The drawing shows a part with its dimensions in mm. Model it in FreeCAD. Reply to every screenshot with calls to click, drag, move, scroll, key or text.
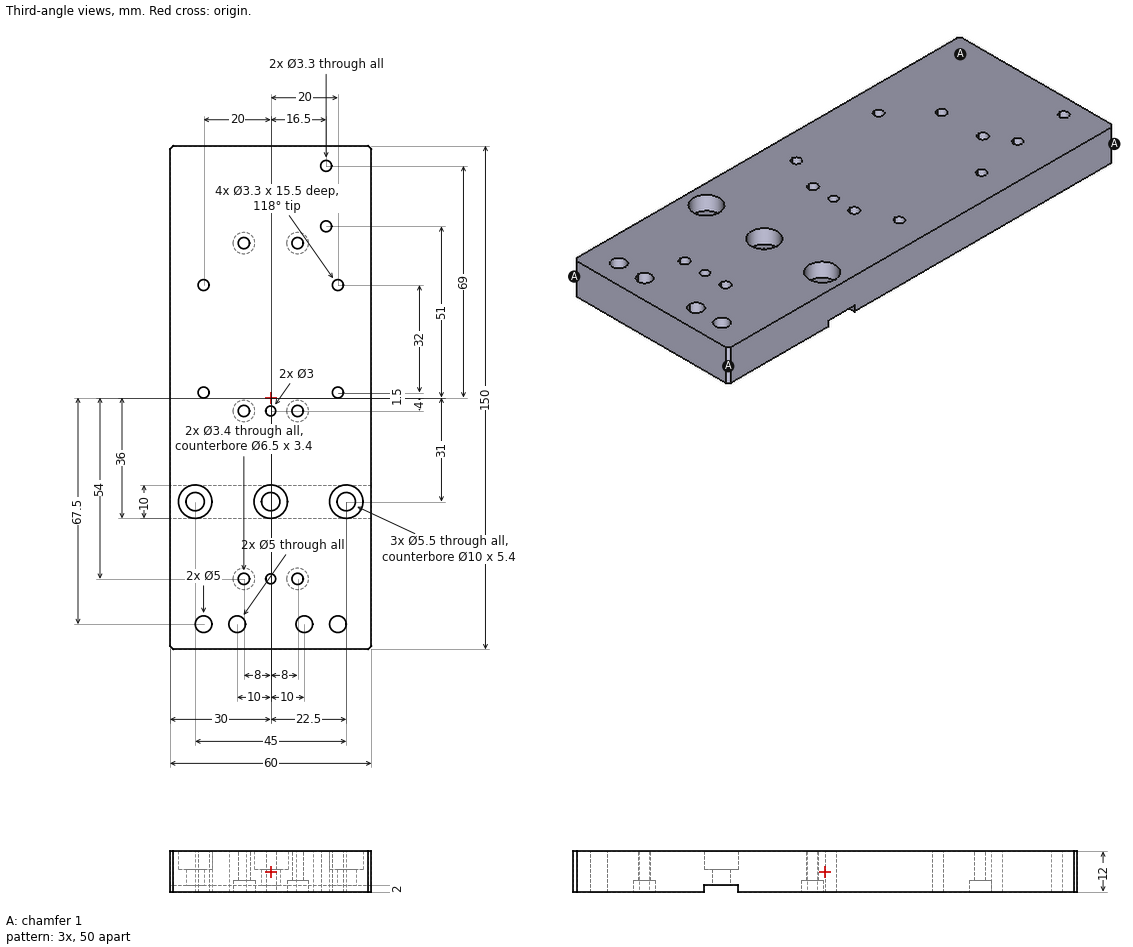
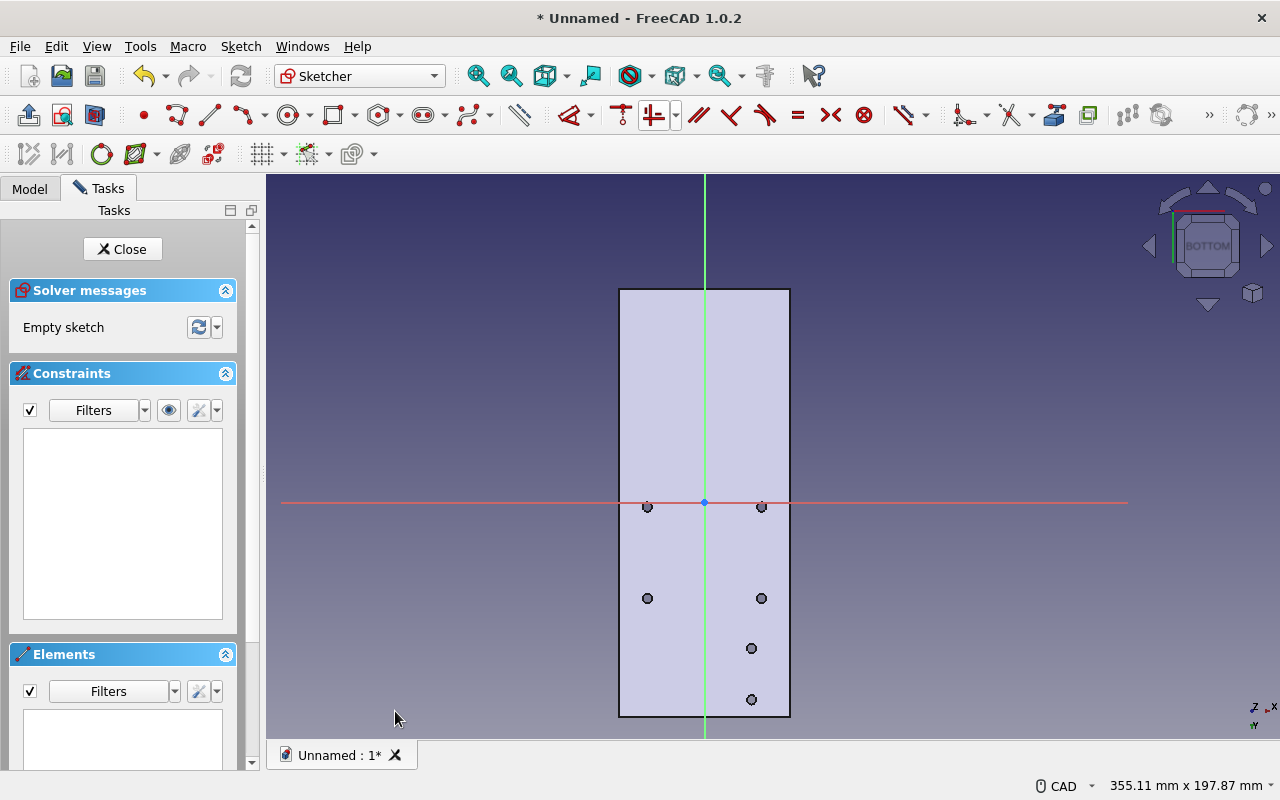
scroll(705, 338, up, 3)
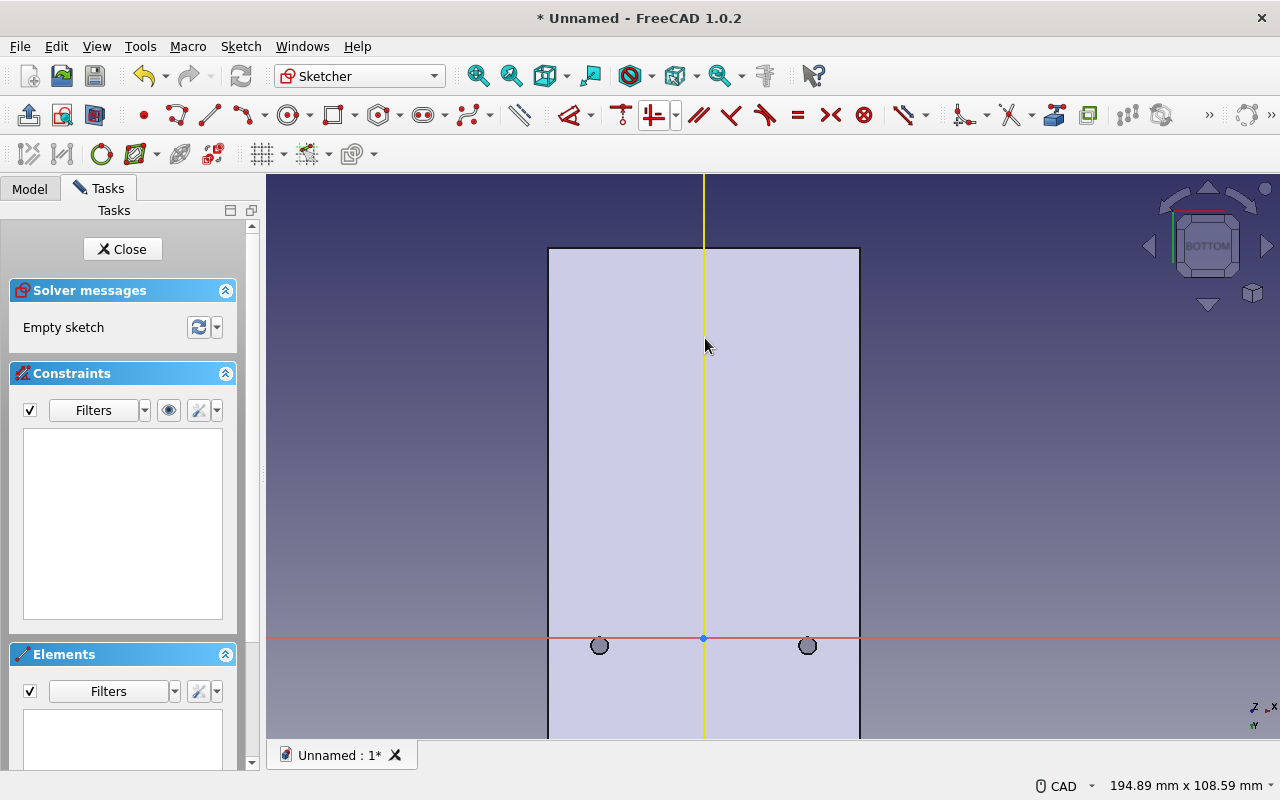
click(288, 116)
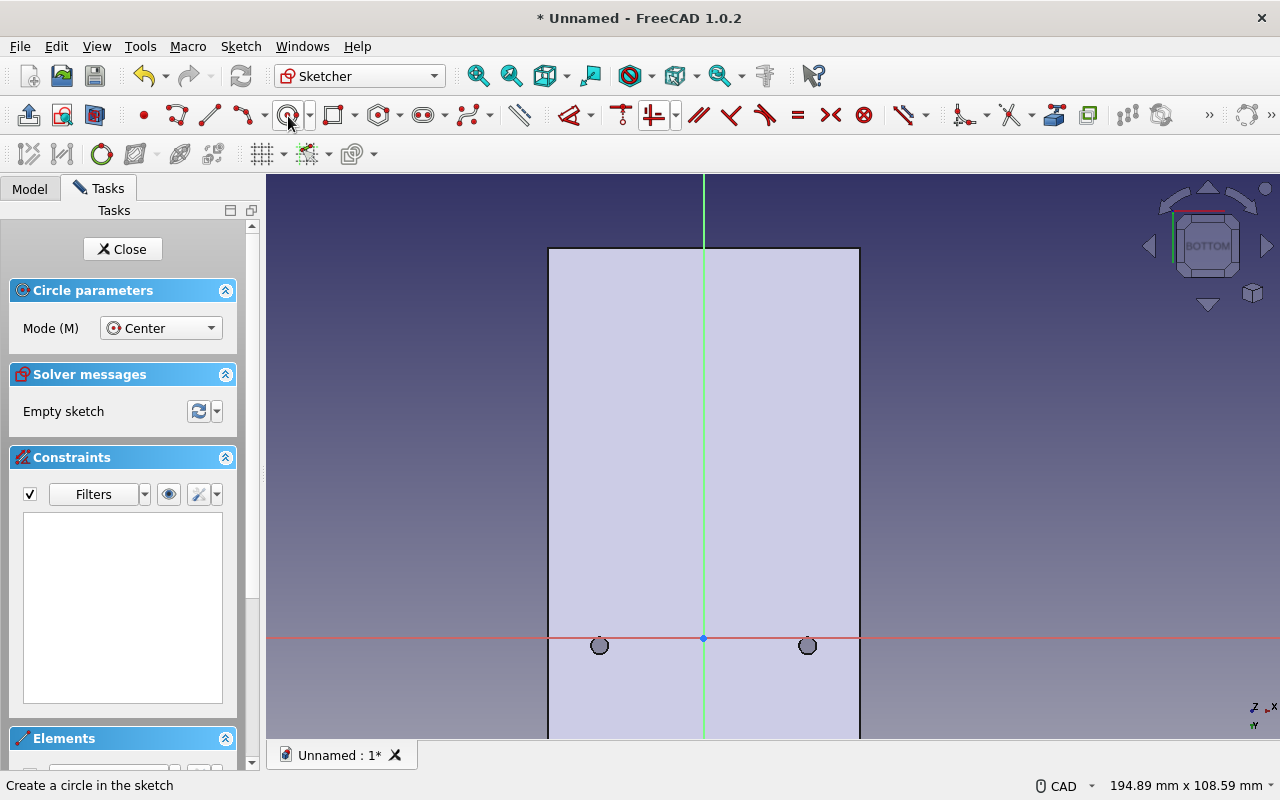
scroll(600, 287, up, 3)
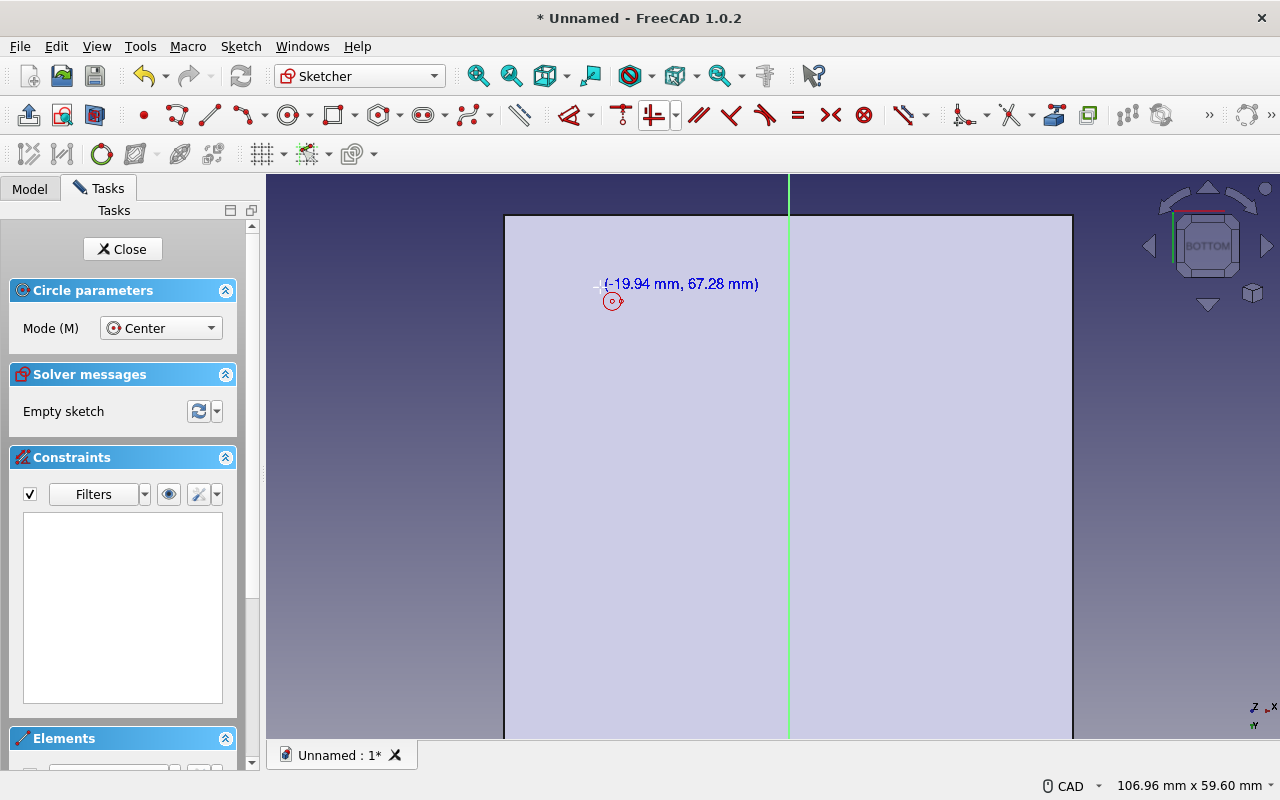
click(599, 287)
click(616, 270)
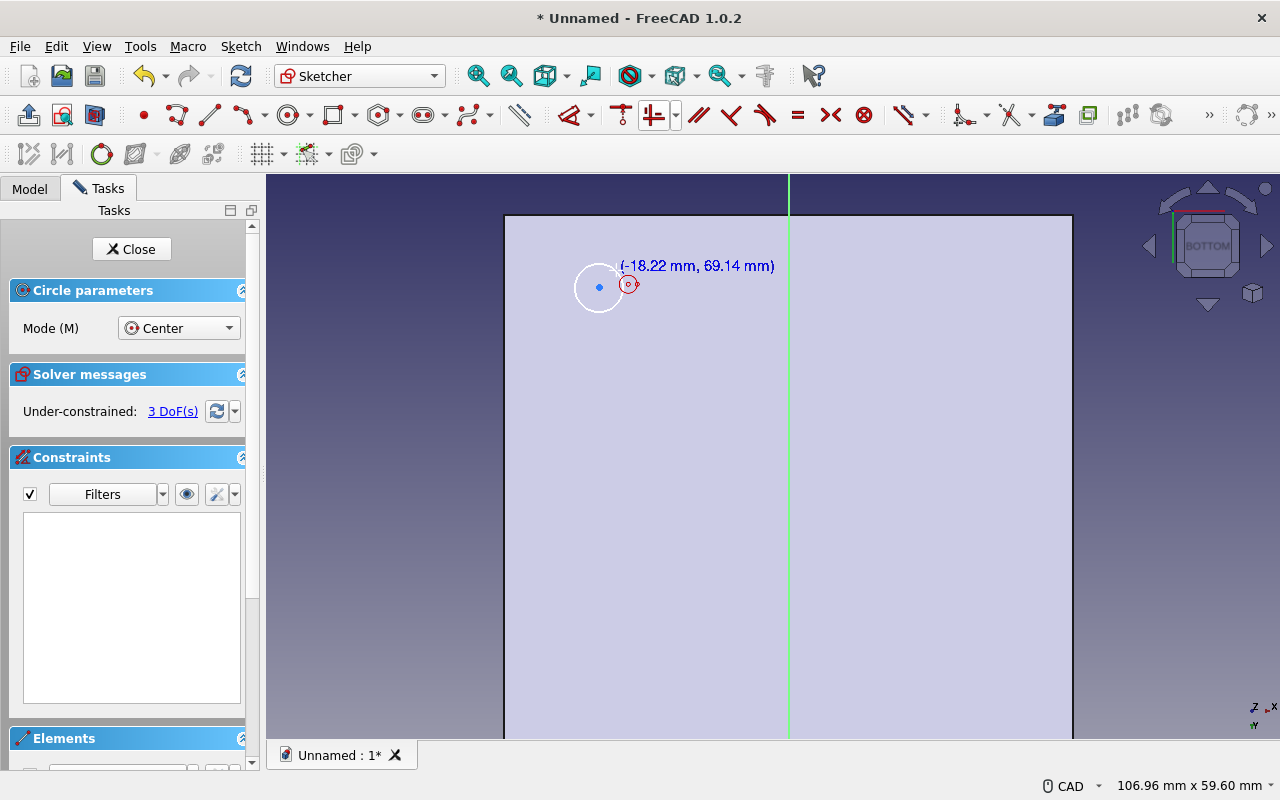
click(978, 287)
click(995, 270)
key(Escape)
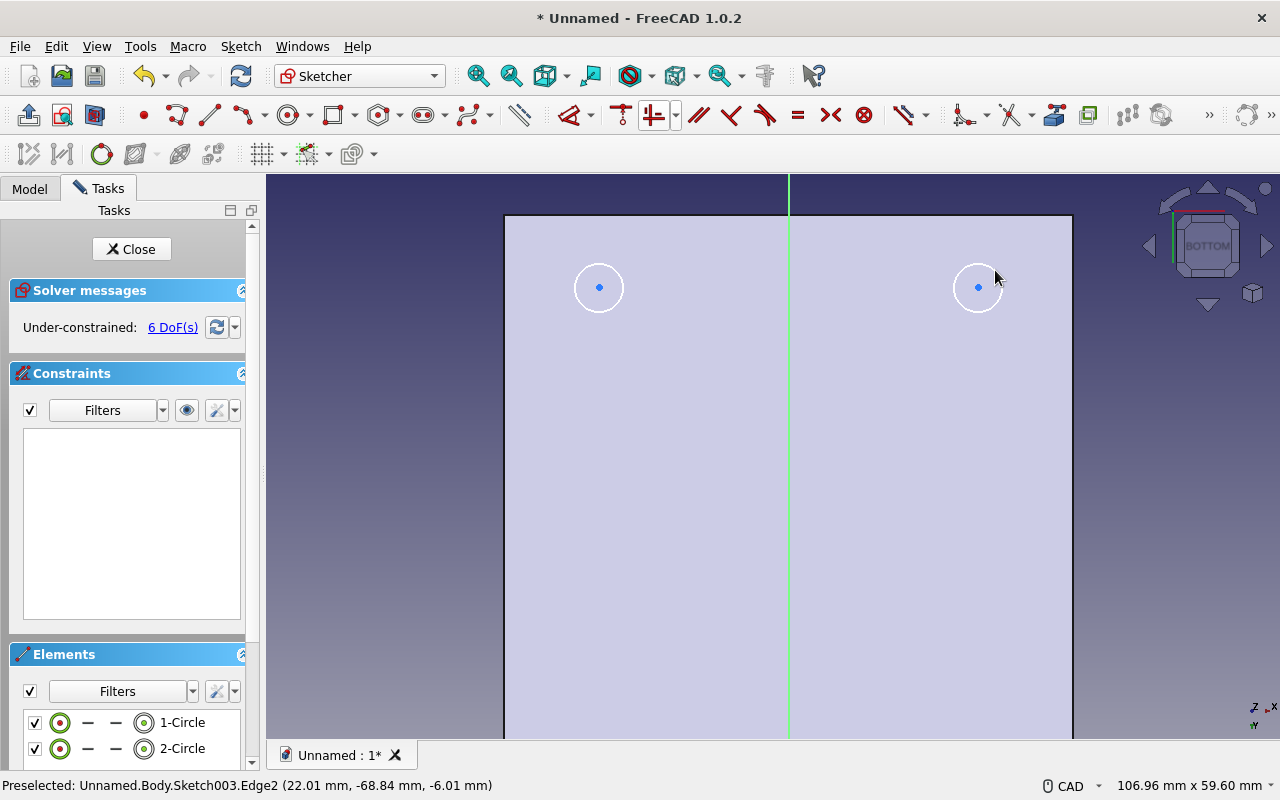
click(616, 271)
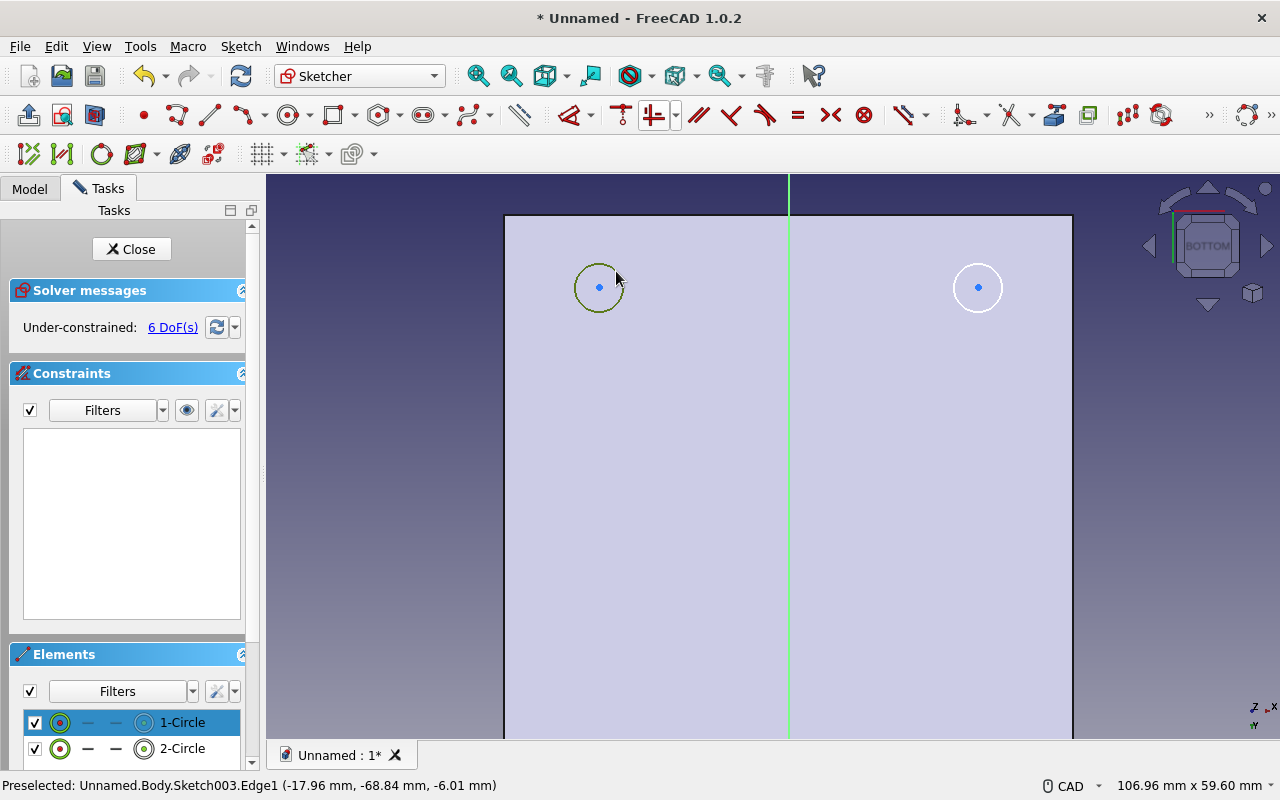
click(995, 271)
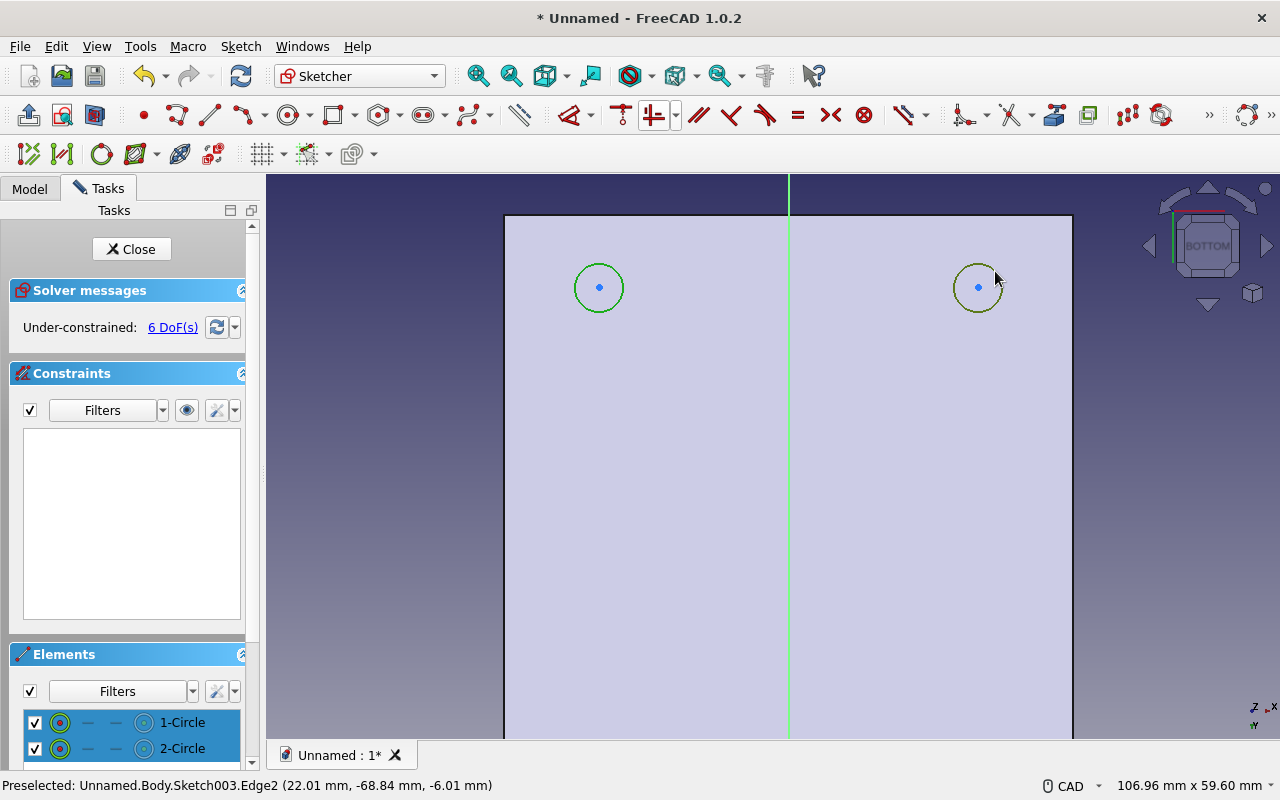
click(798, 116)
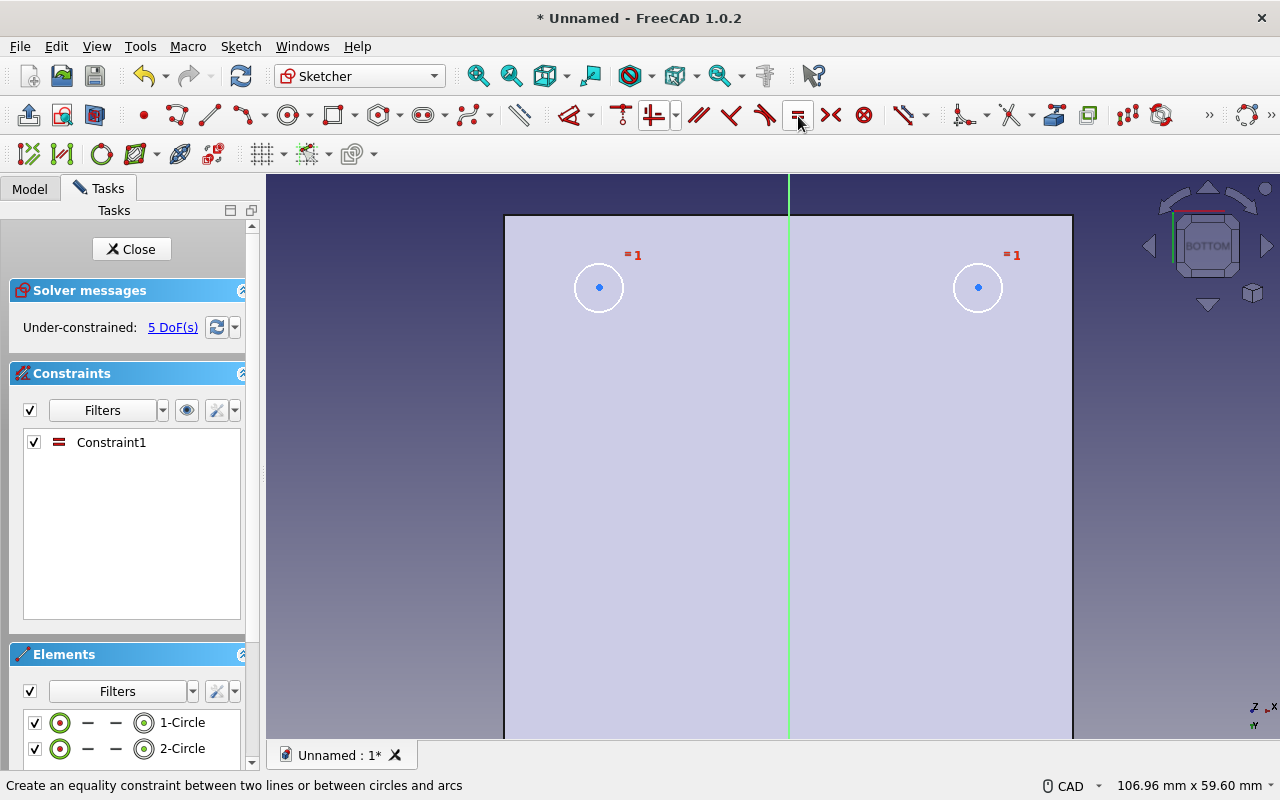
click(599, 288)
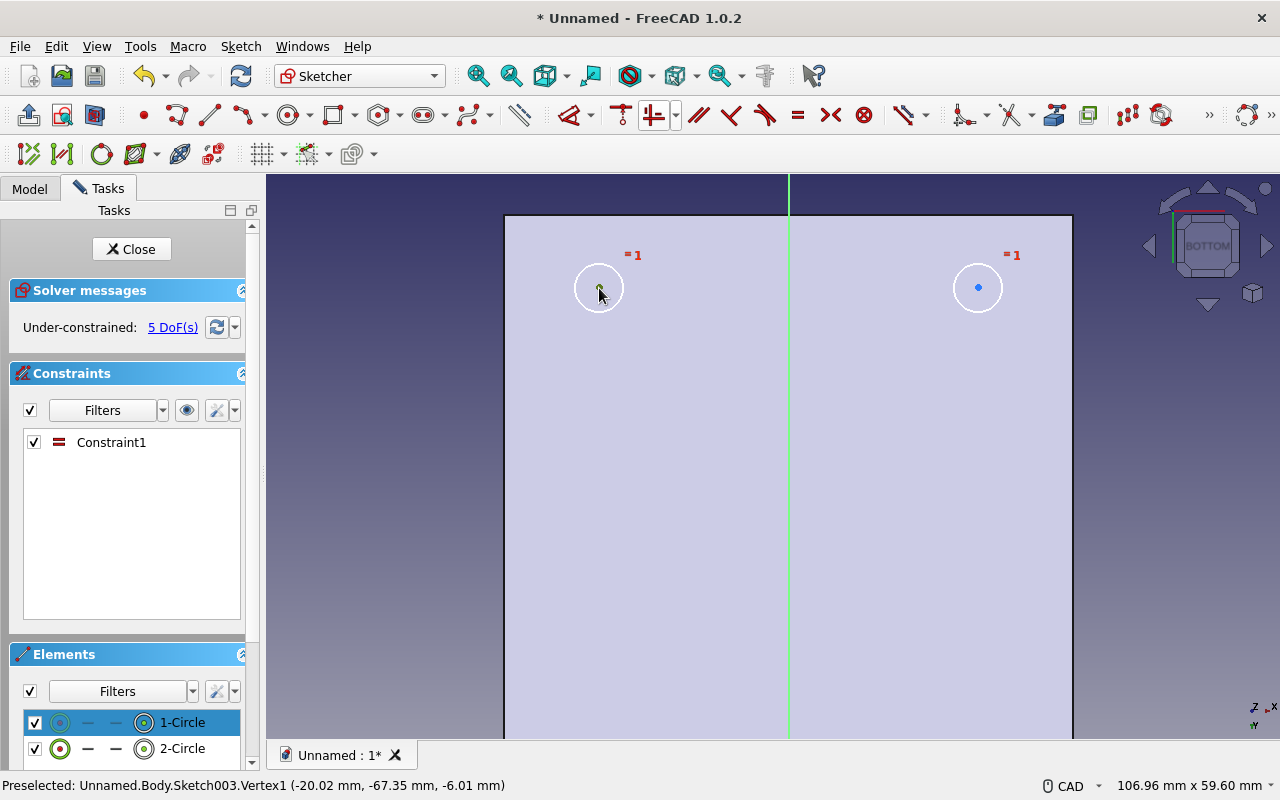
click(978, 288)